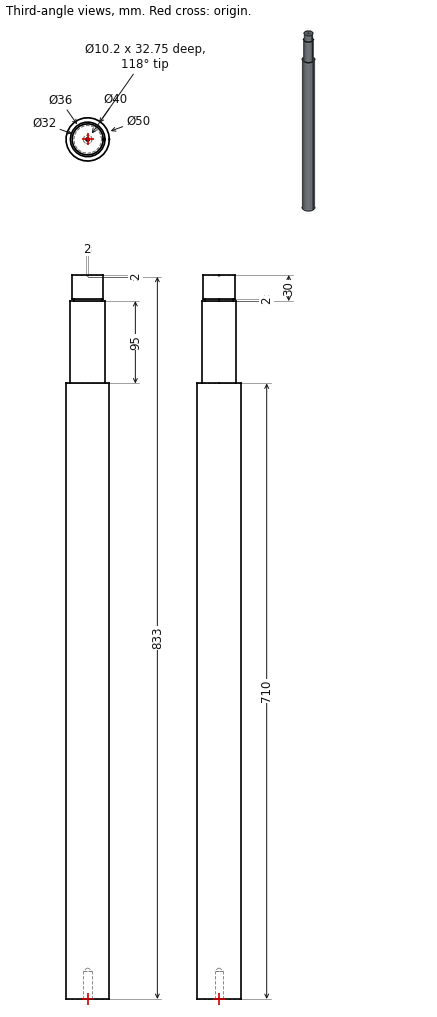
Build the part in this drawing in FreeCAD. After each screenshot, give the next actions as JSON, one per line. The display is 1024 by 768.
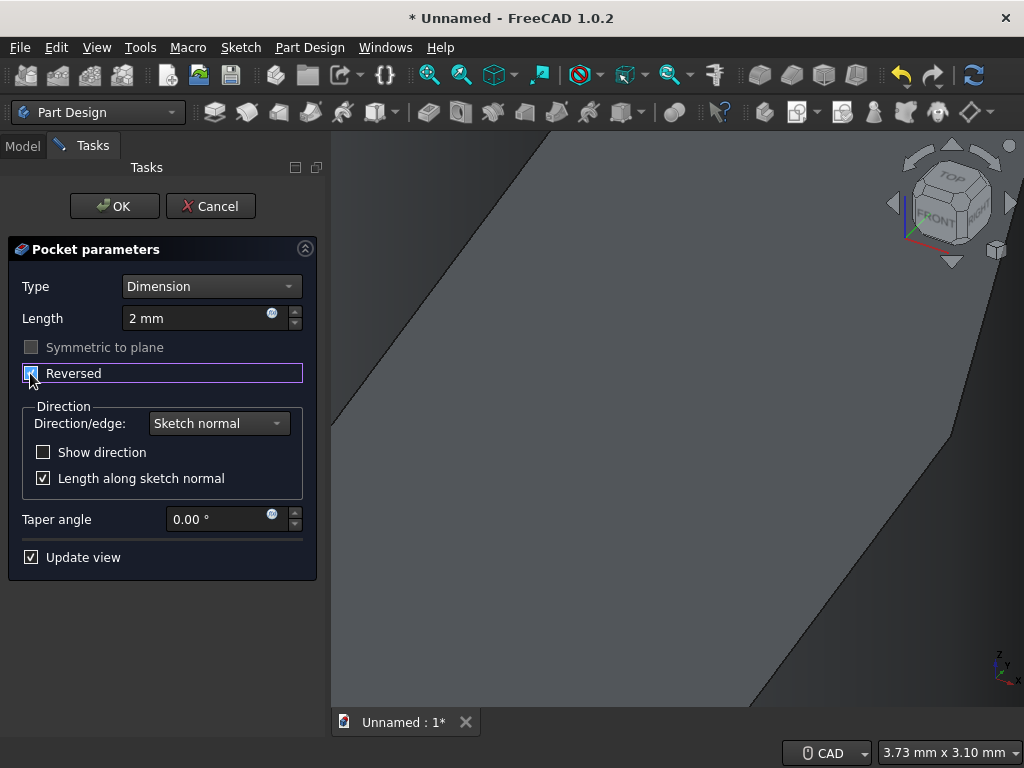
{"action": "left_click", "coordinate": [115, 206]}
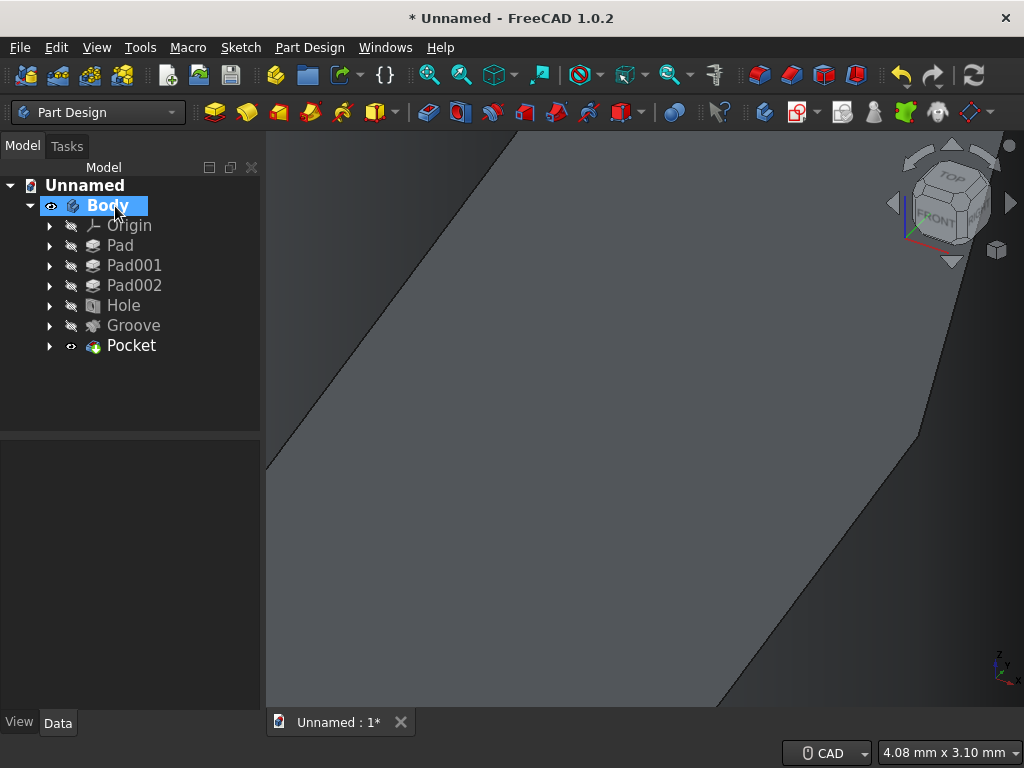
{"action": "key", "text": "0"}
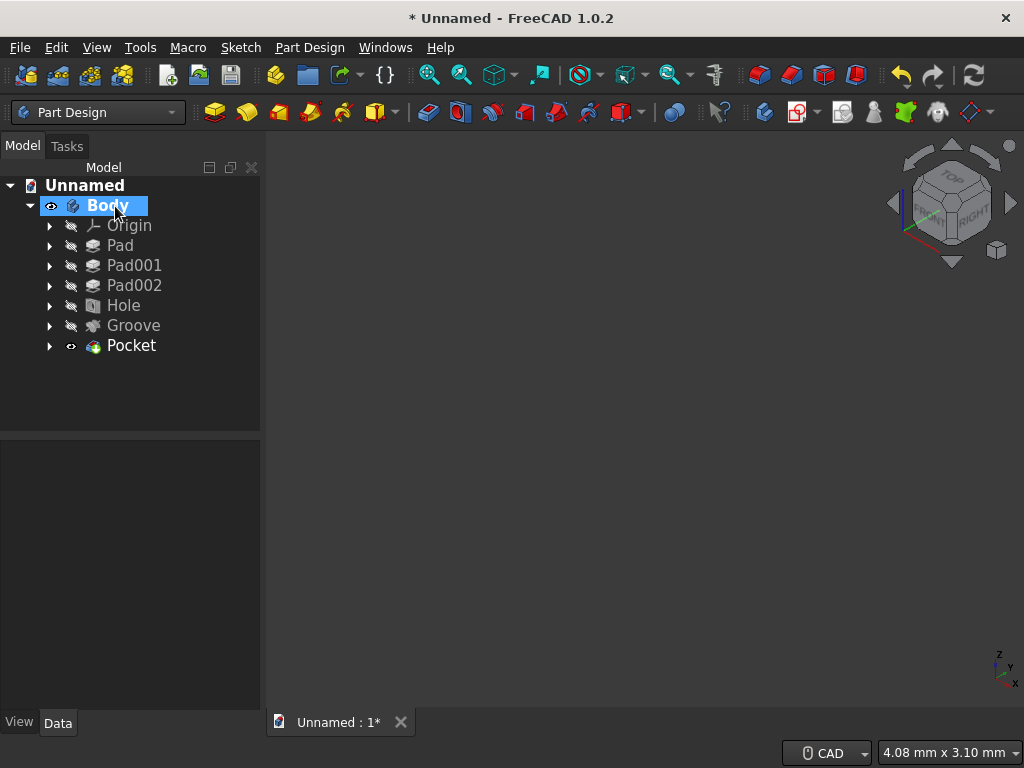
{"action": "left_click", "coordinate": [430, 76]}